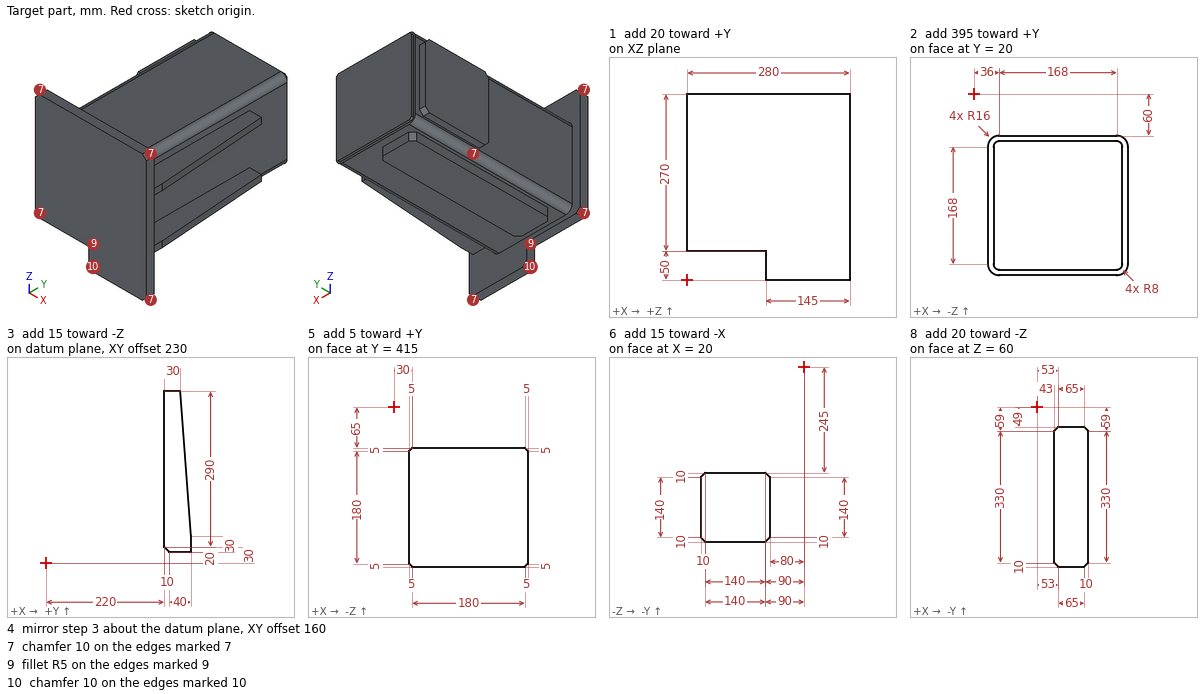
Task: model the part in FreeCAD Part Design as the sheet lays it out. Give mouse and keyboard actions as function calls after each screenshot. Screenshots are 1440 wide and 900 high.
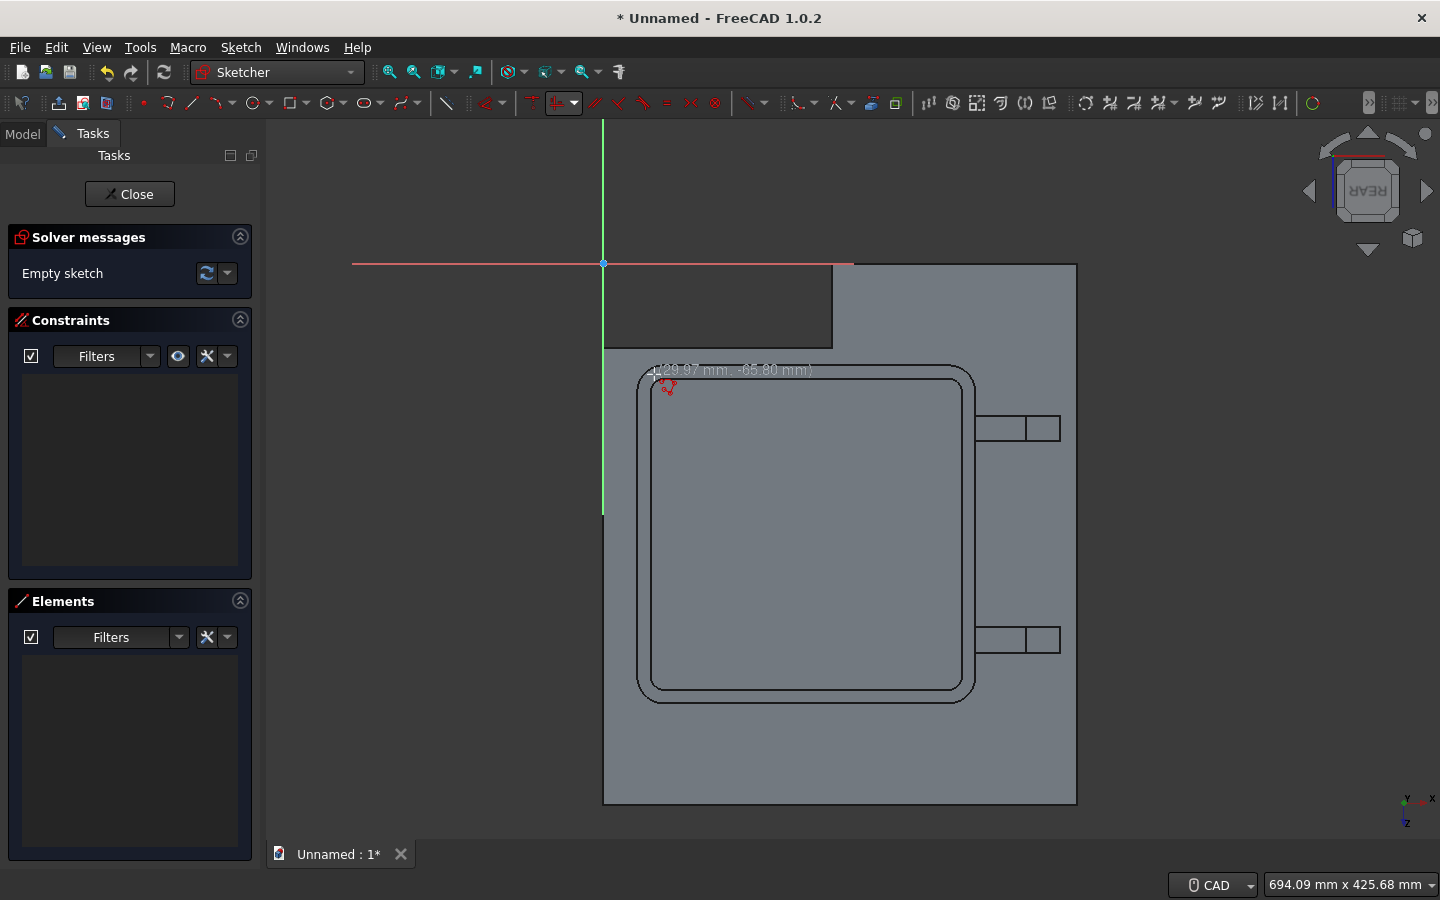
scroll(646, 382, up, 2)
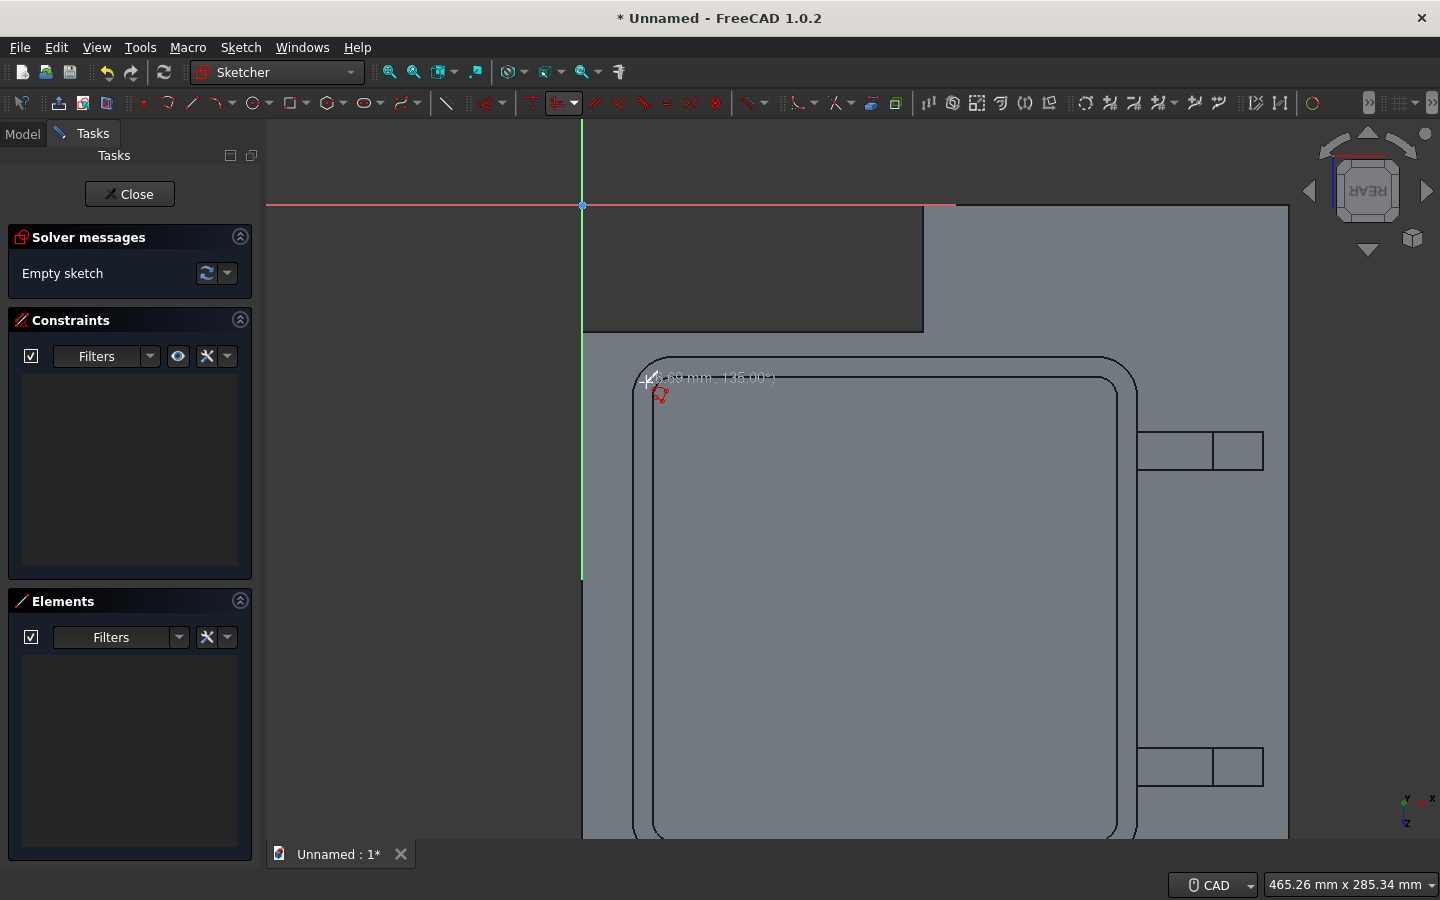
click(645, 382)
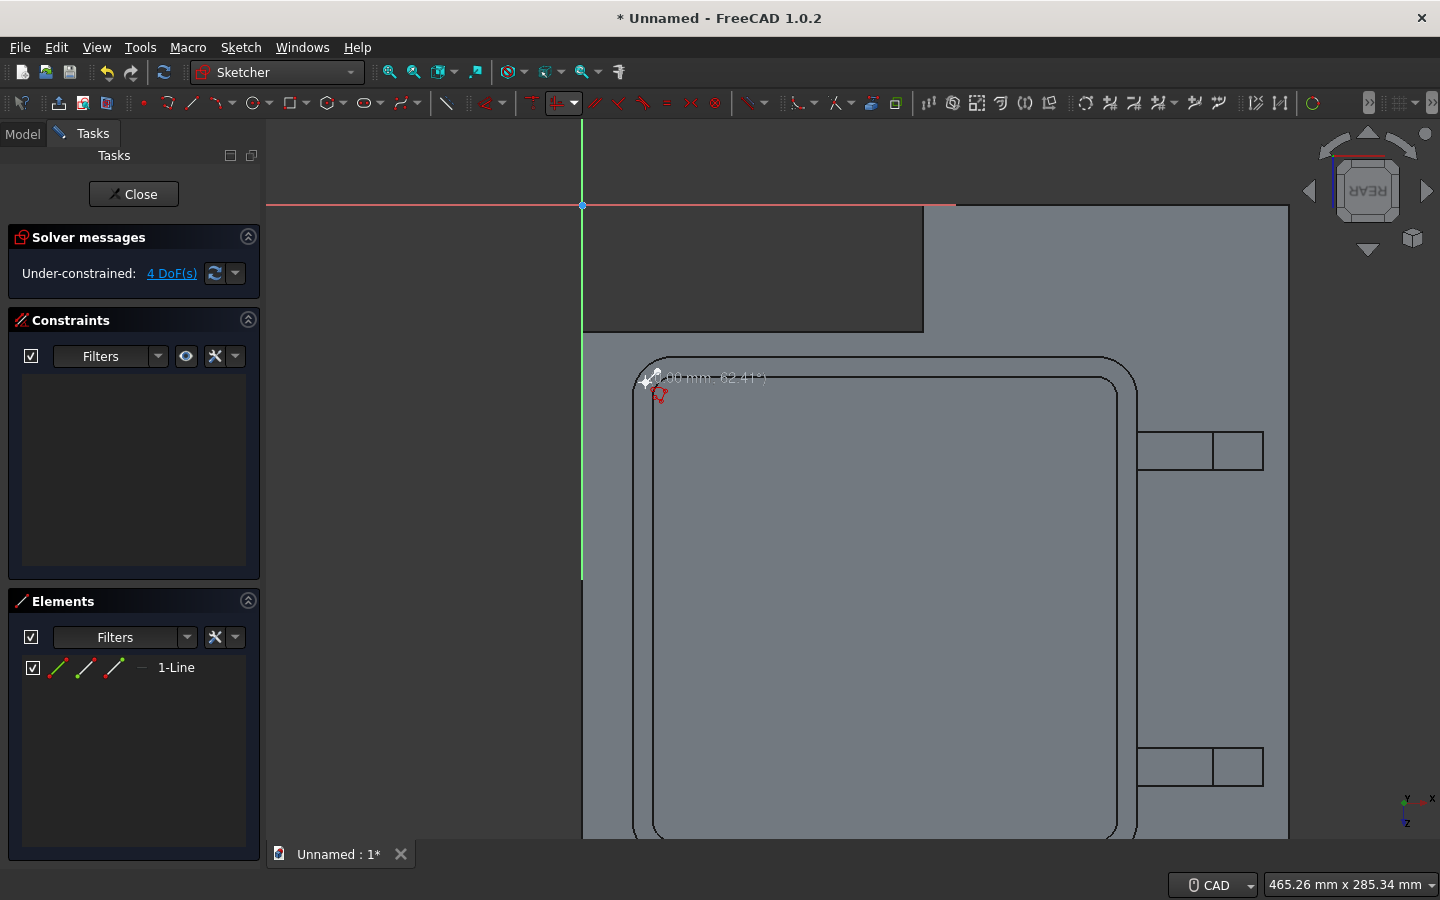
scroll(644, 381, down, 2)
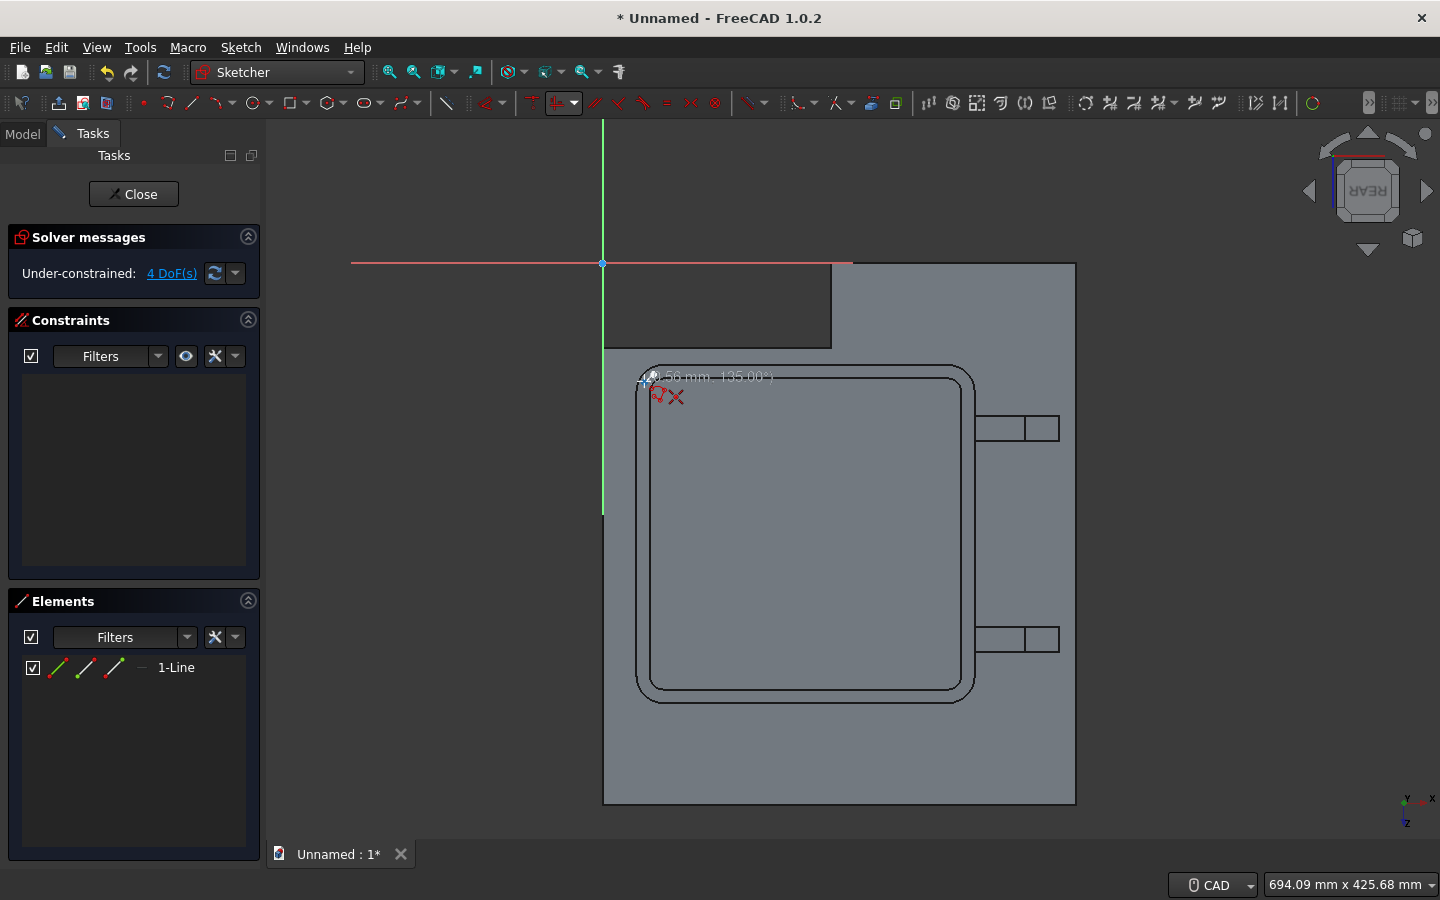
click(645, 686)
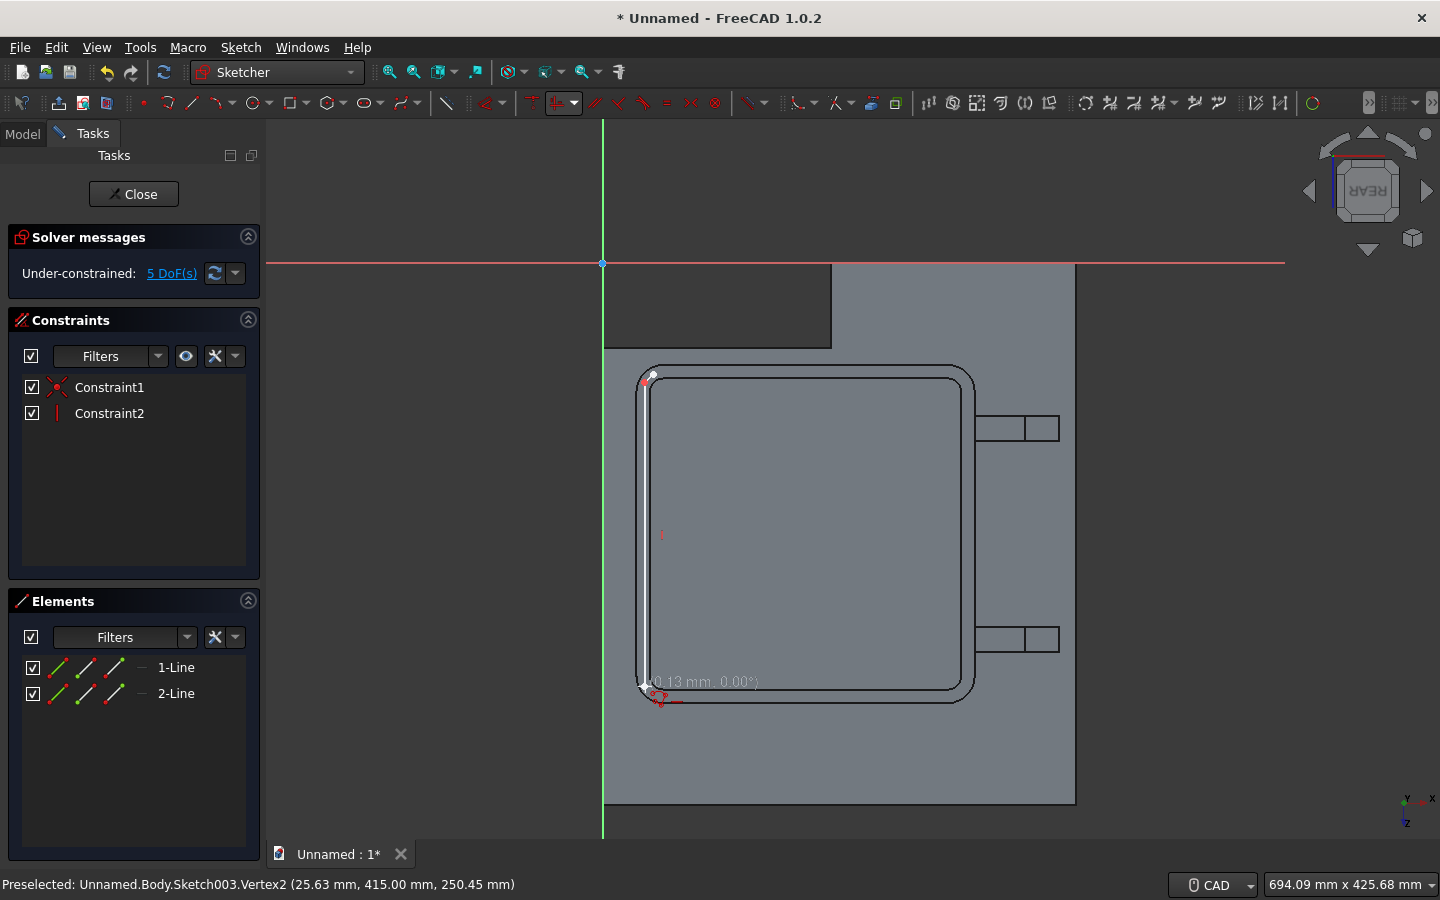
scroll(653, 695, up, 2)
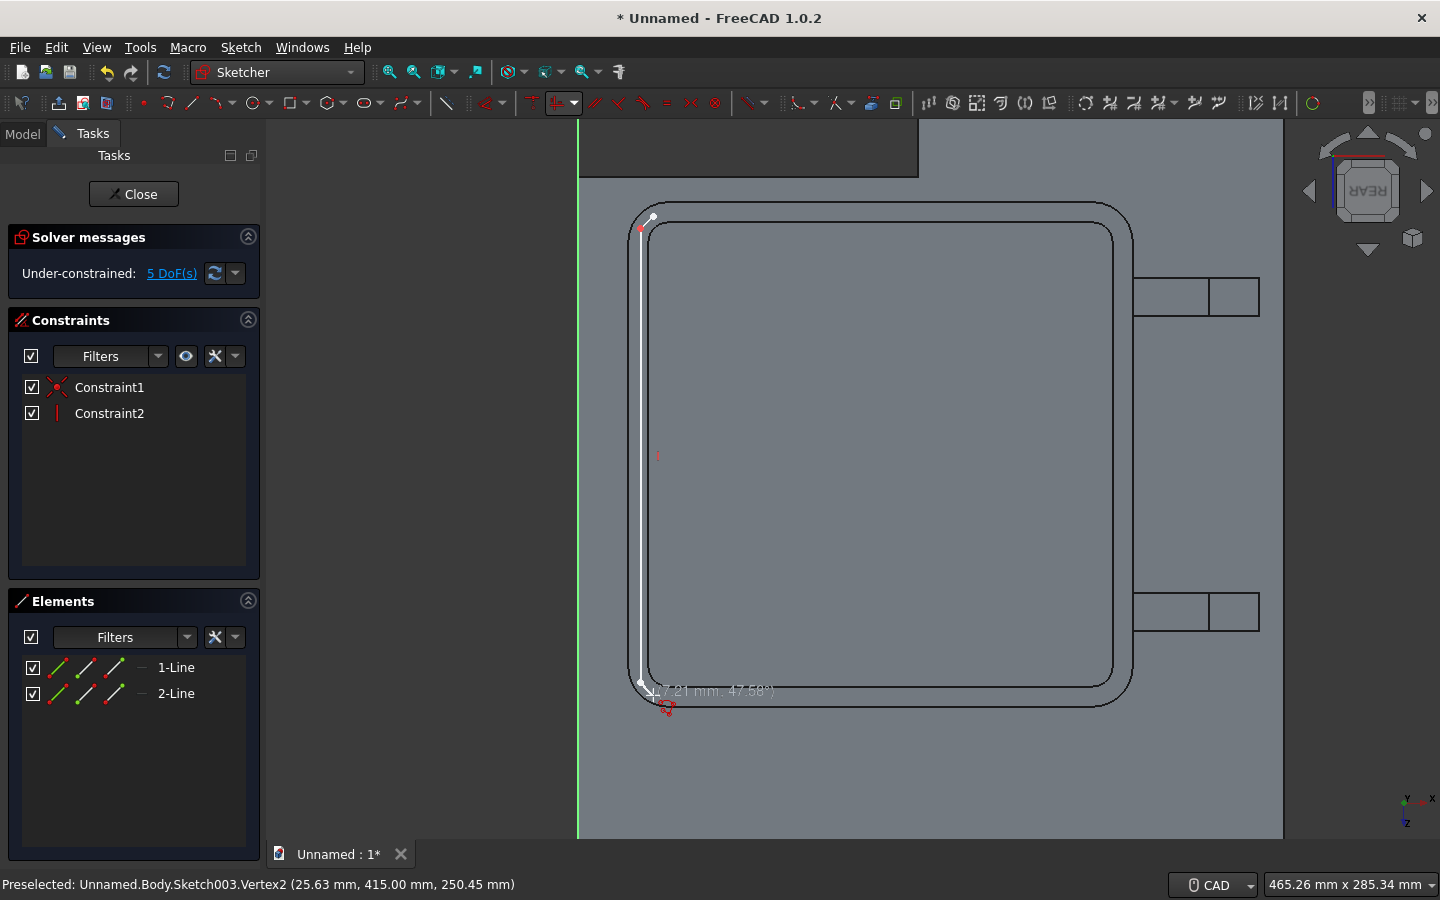
click(653, 694)
click(1108, 694)
click(1120, 682)
click(1120, 227)
click(1108, 215)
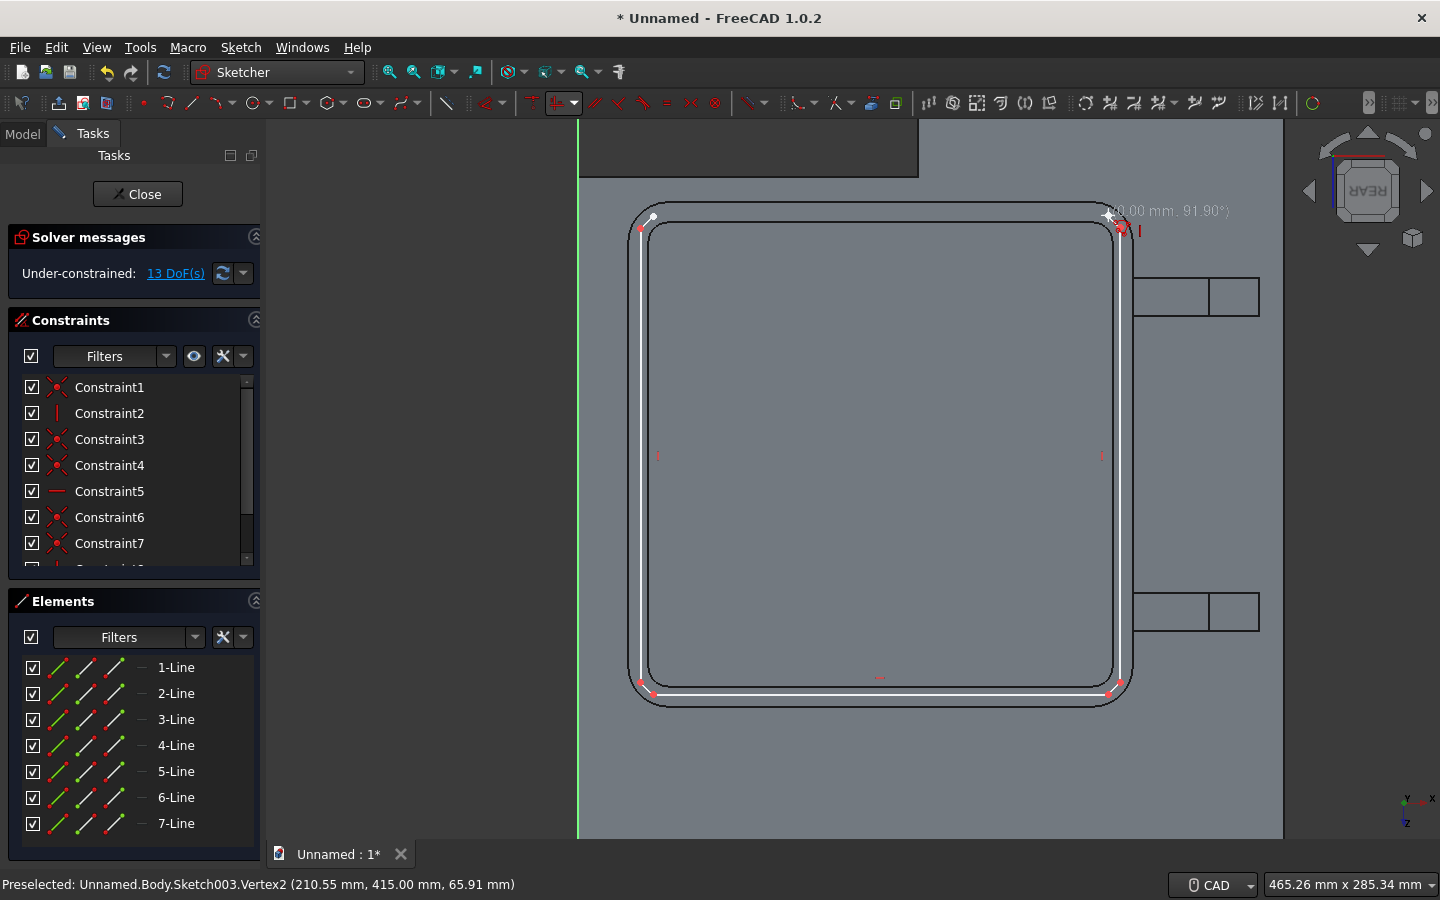
scroll(653, 215, up, 3)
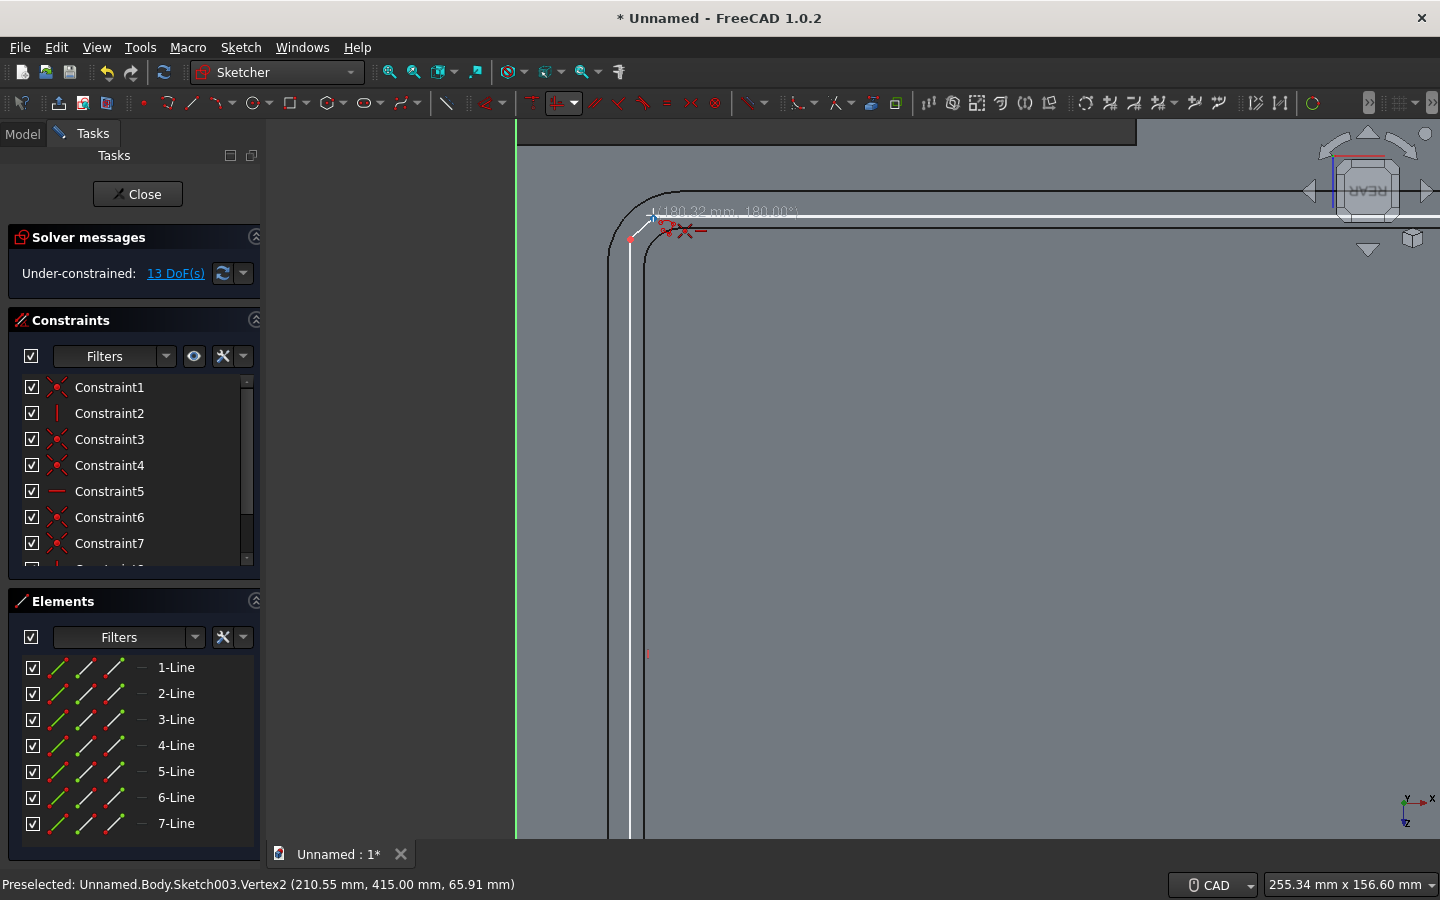
click(653, 218)
key(Escape)
key(Escape)